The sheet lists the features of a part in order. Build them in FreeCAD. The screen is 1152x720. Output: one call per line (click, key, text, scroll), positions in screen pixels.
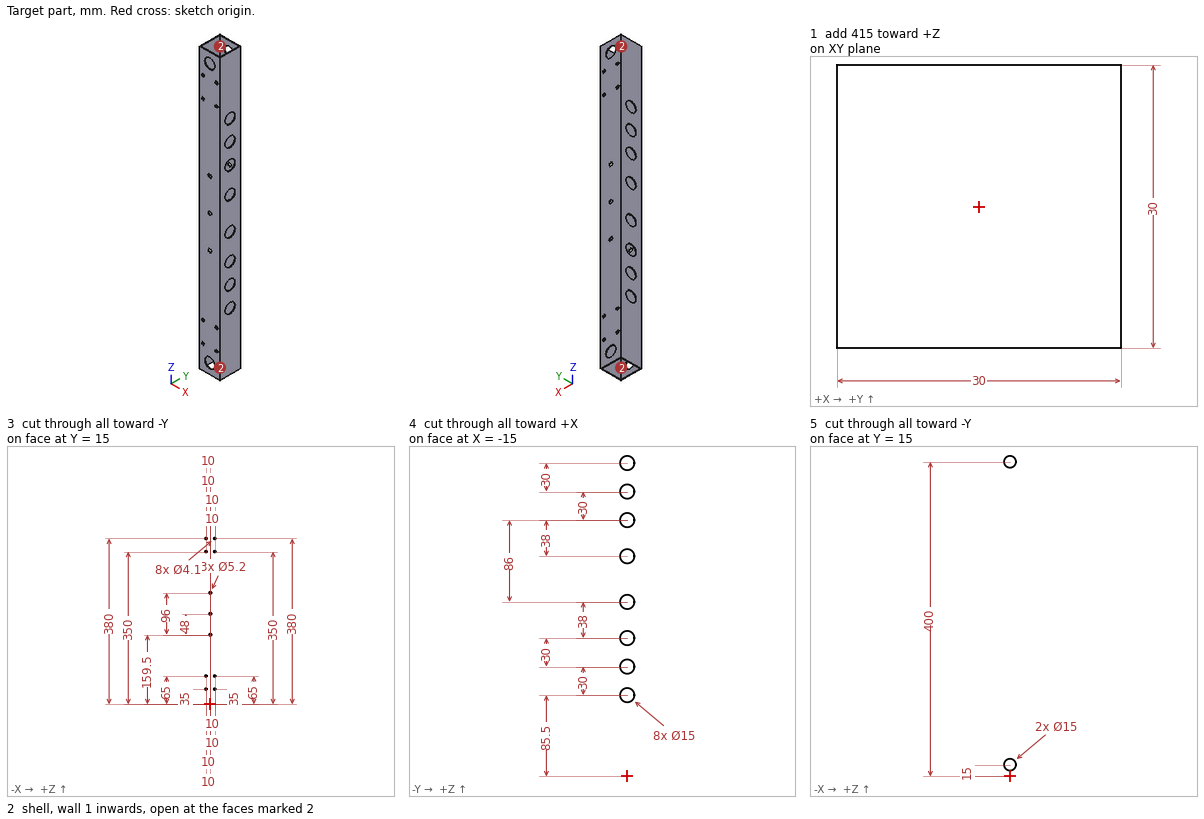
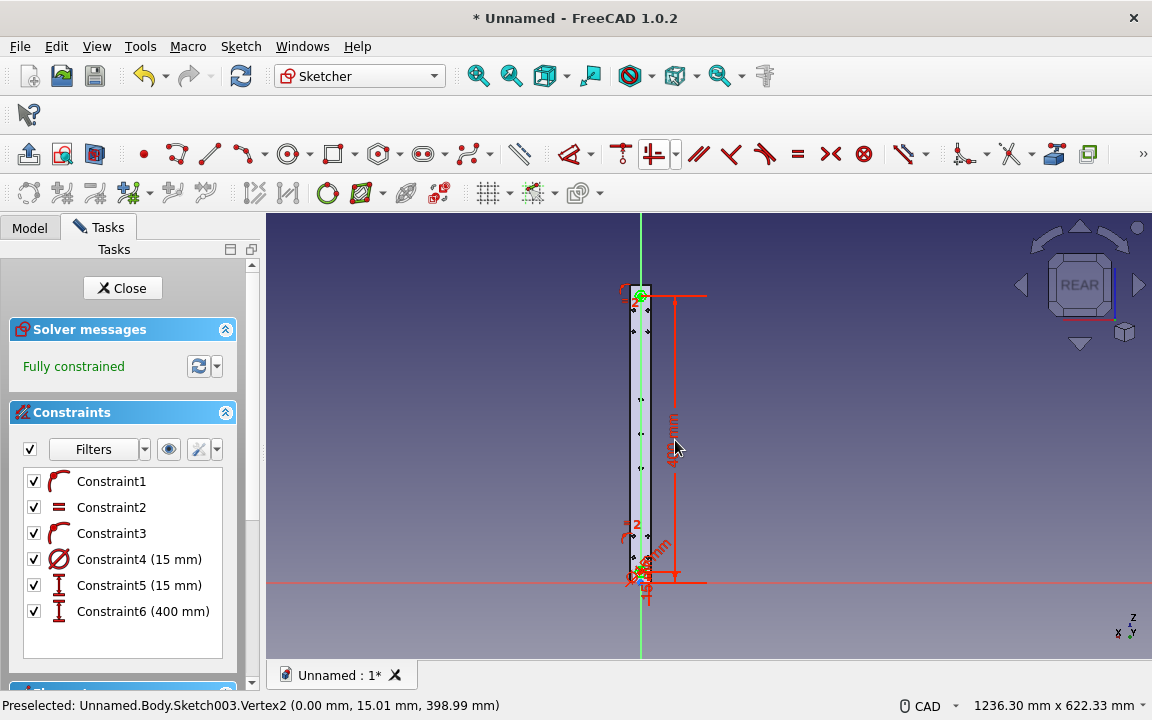
click(123, 288)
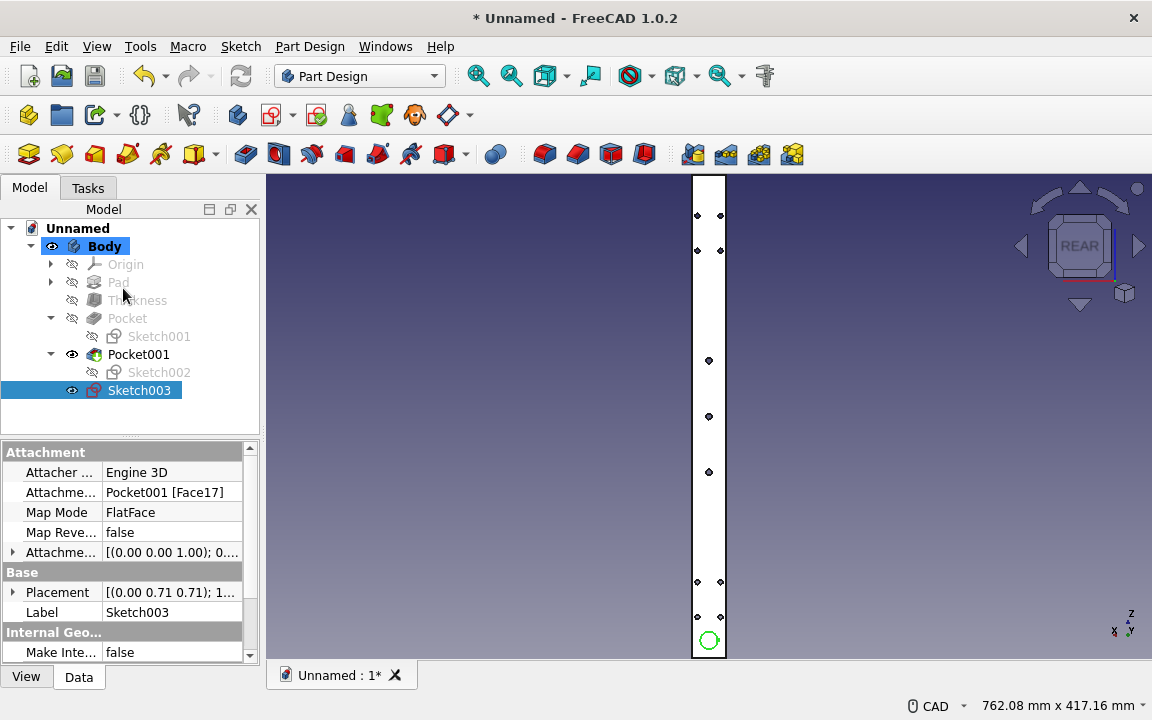
click(246, 154)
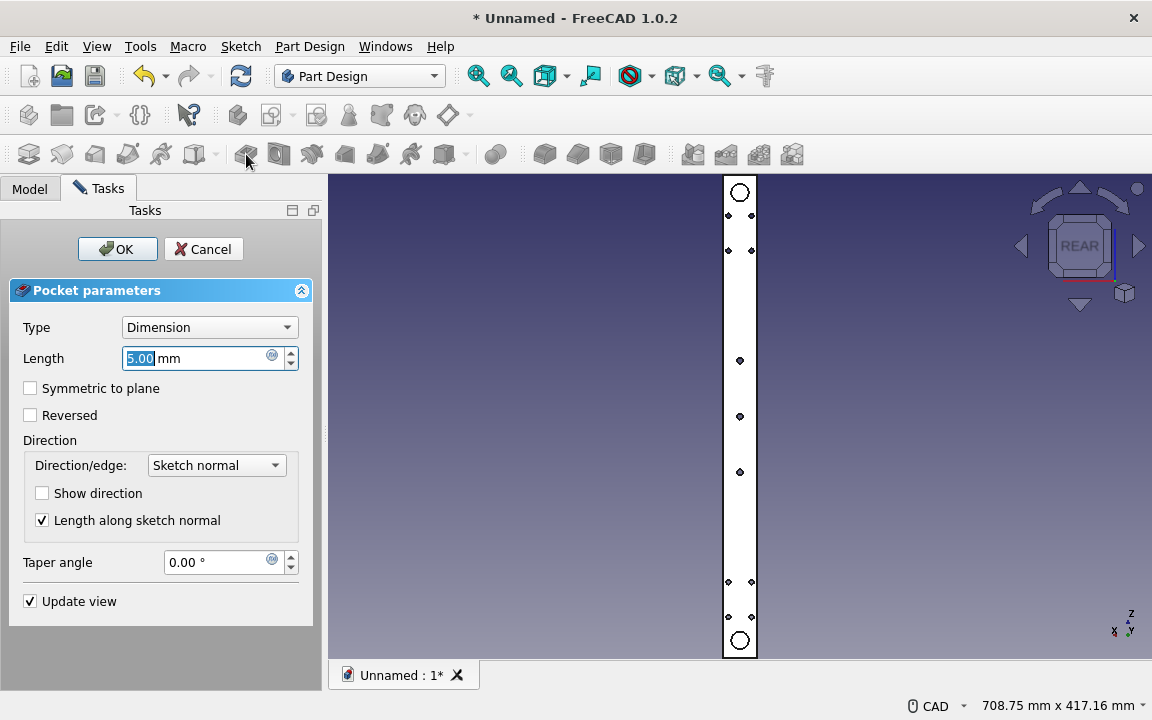
click(210, 328)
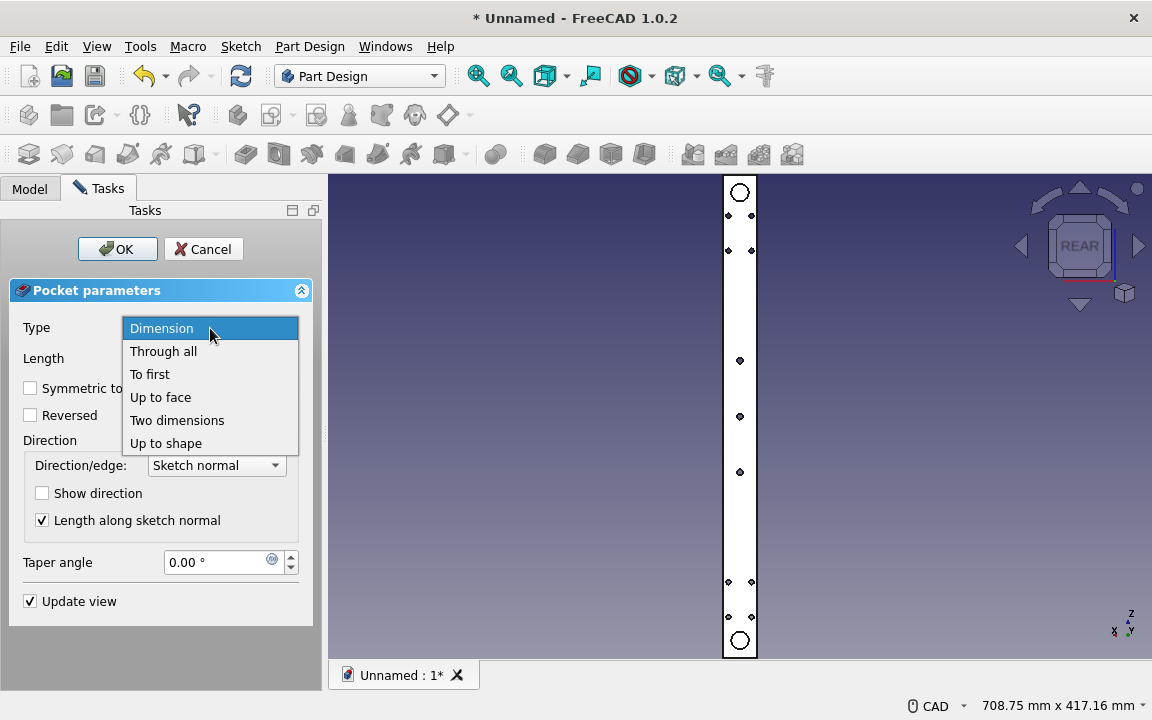
click(208, 352)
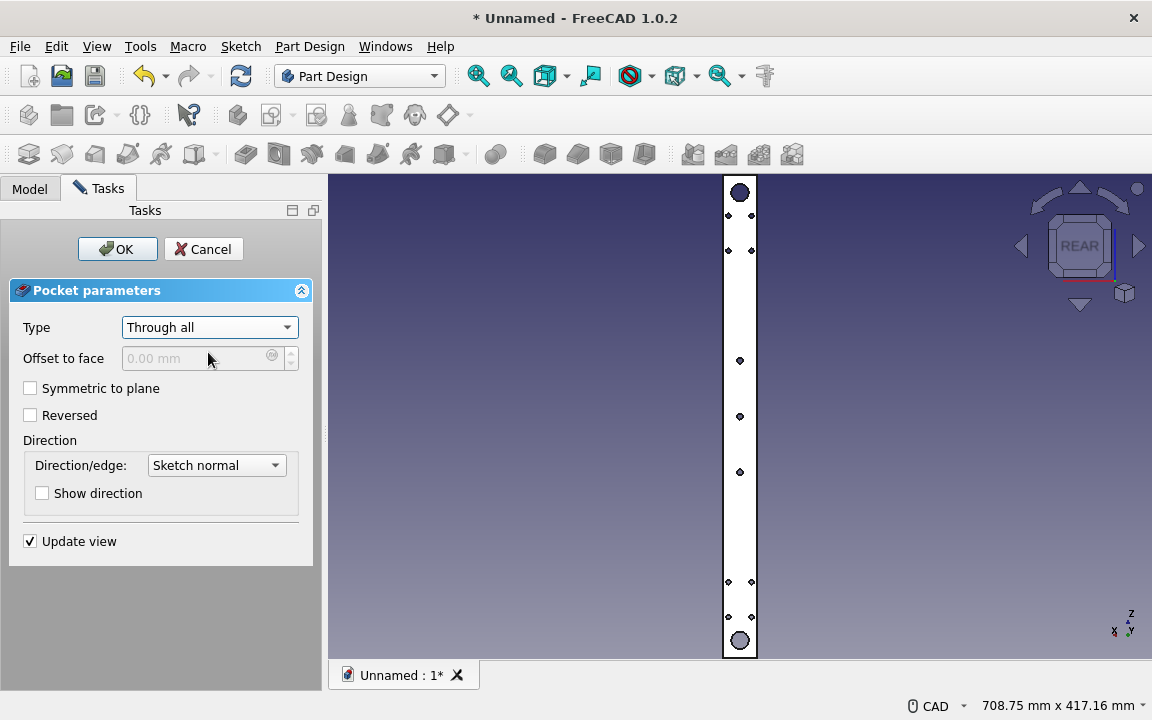
click(118, 249)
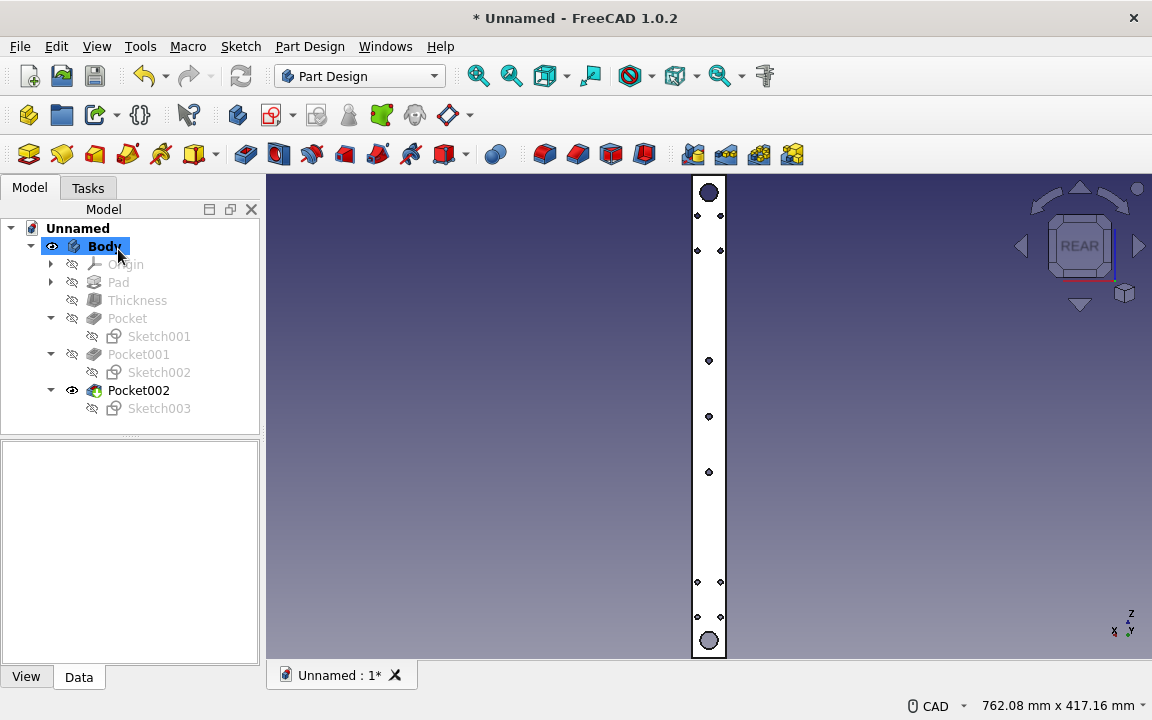
key(0)